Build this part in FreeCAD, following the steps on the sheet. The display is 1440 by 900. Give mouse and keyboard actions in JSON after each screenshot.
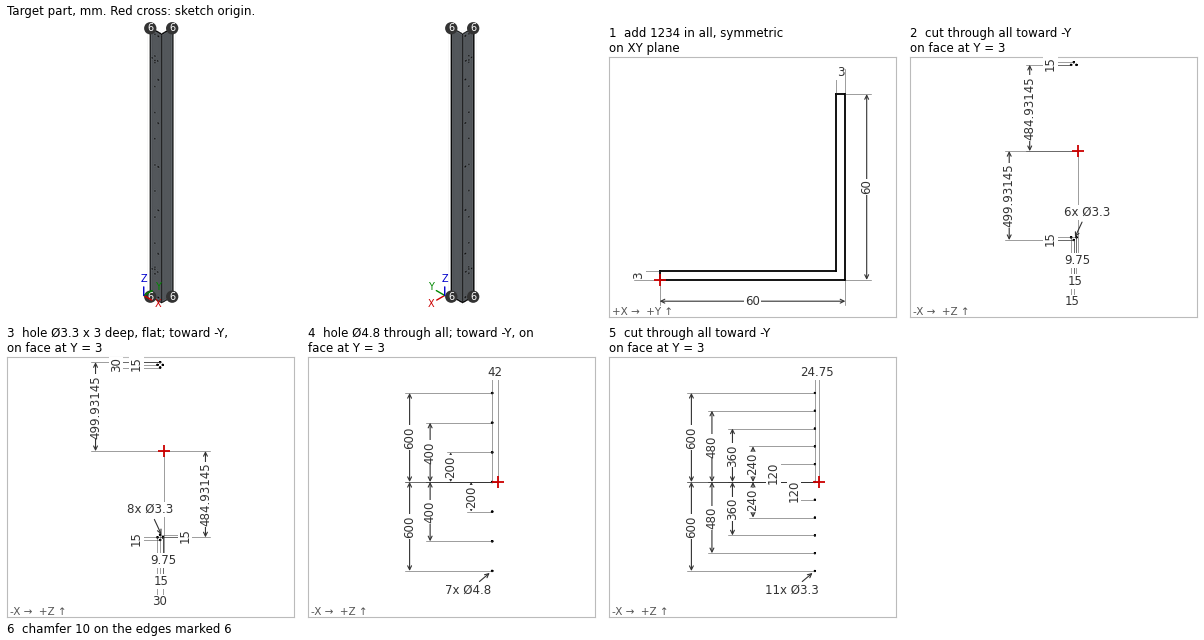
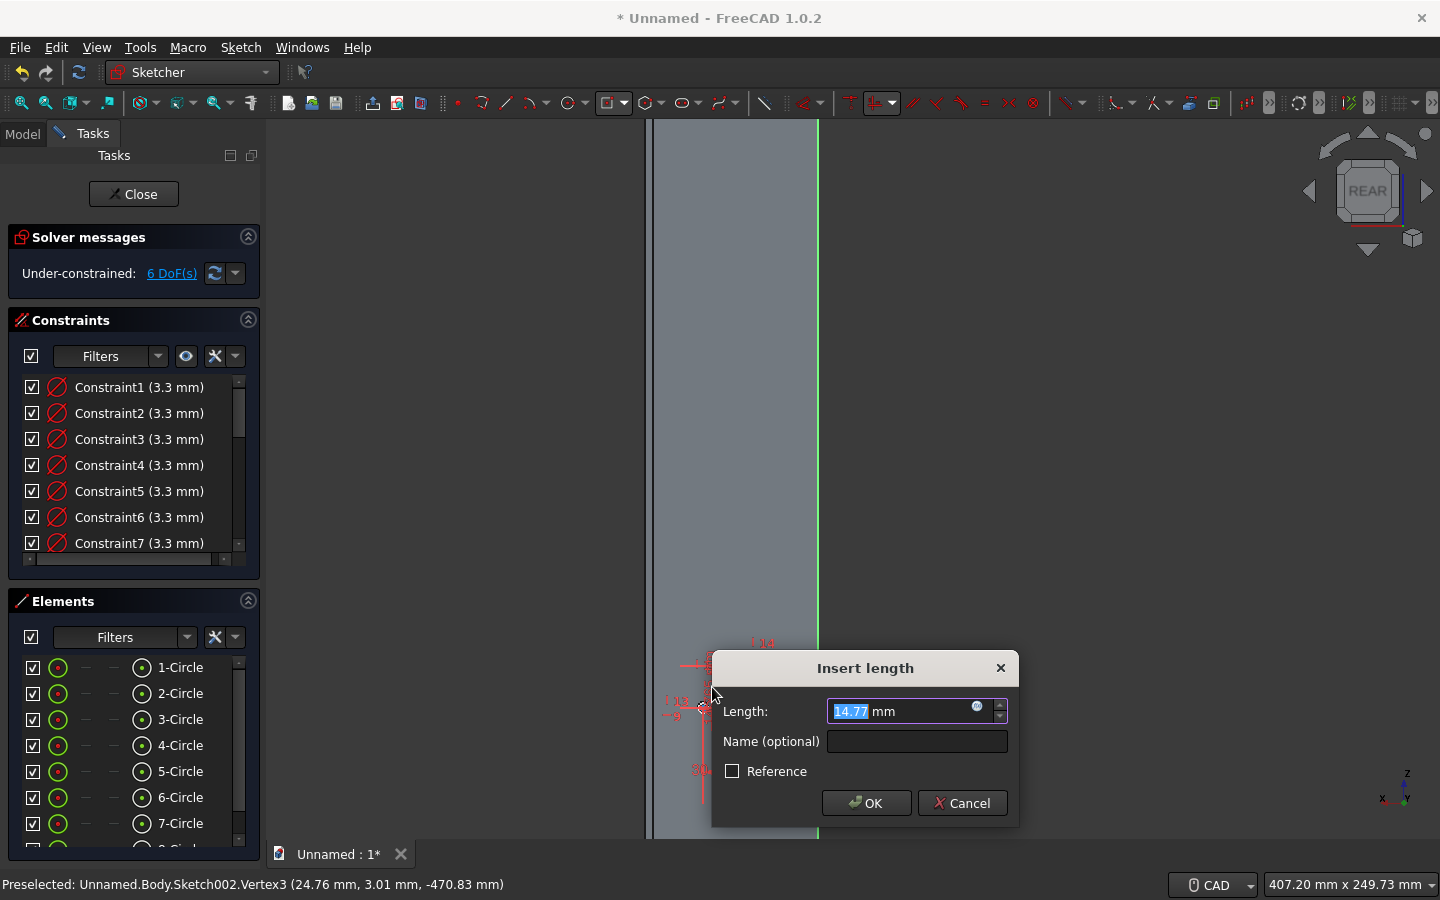
{"action": "type", "text": "15"}
{"action": "key", "text": "Return"}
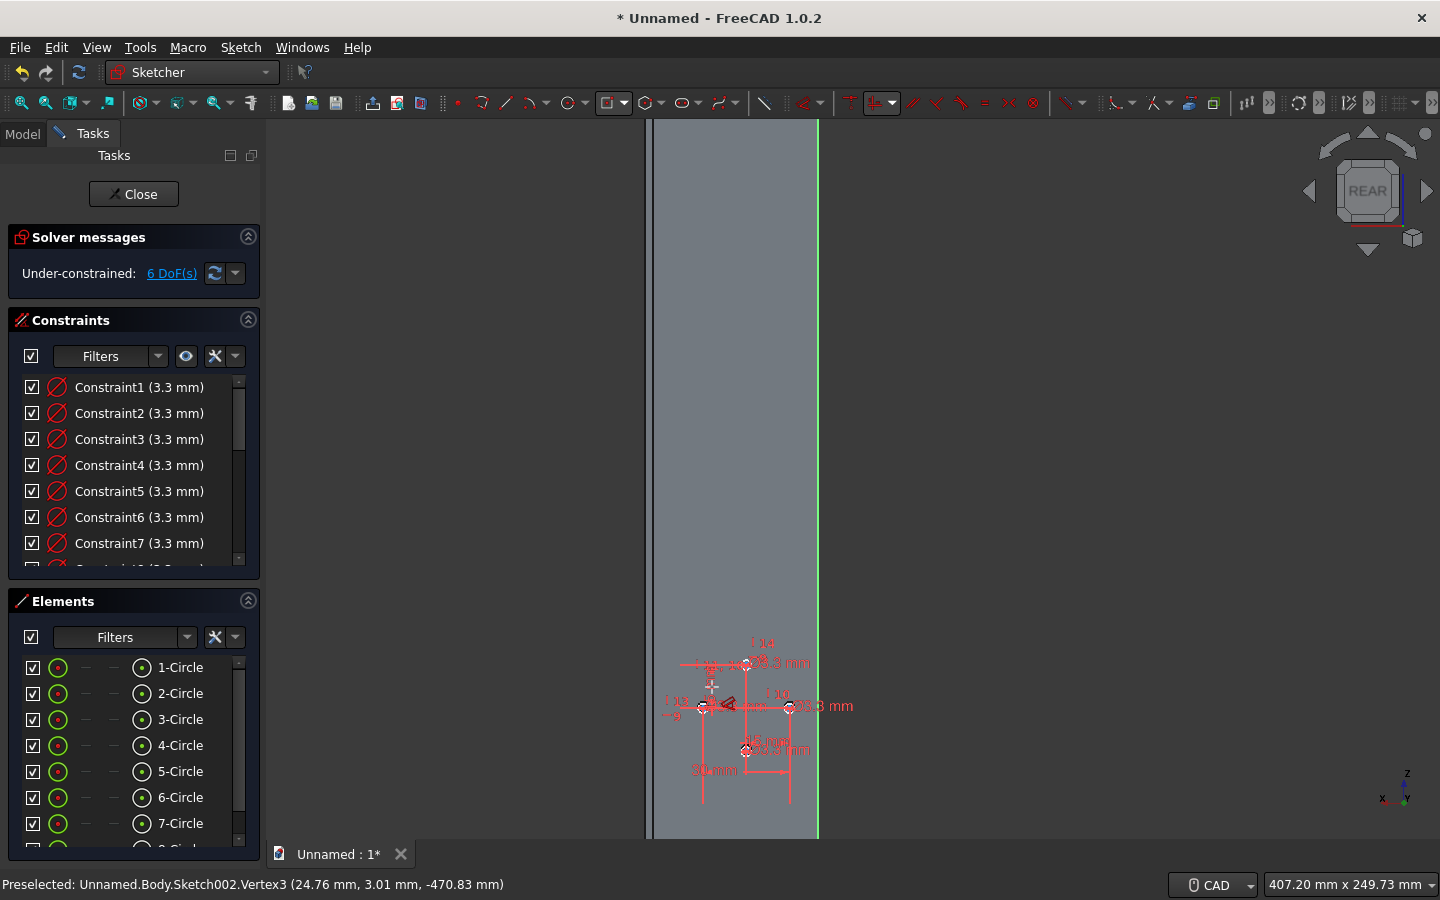
{"action": "left_click", "coordinate": [790, 708]}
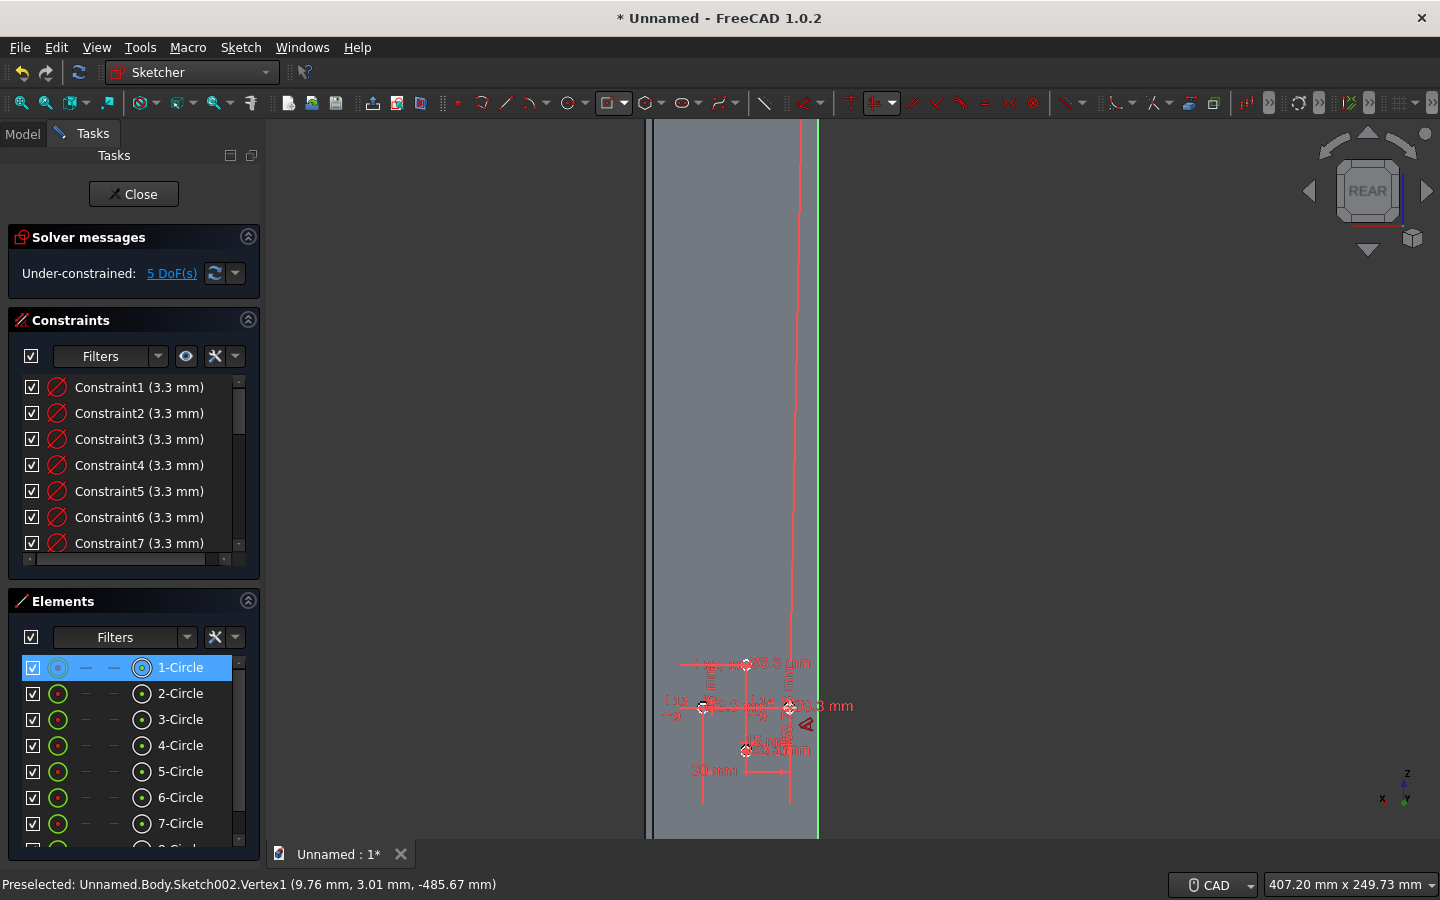
{"action": "left_click", "coordinate": [746, 752]}
{"action": "left_click", "coordinate": [848, 730]}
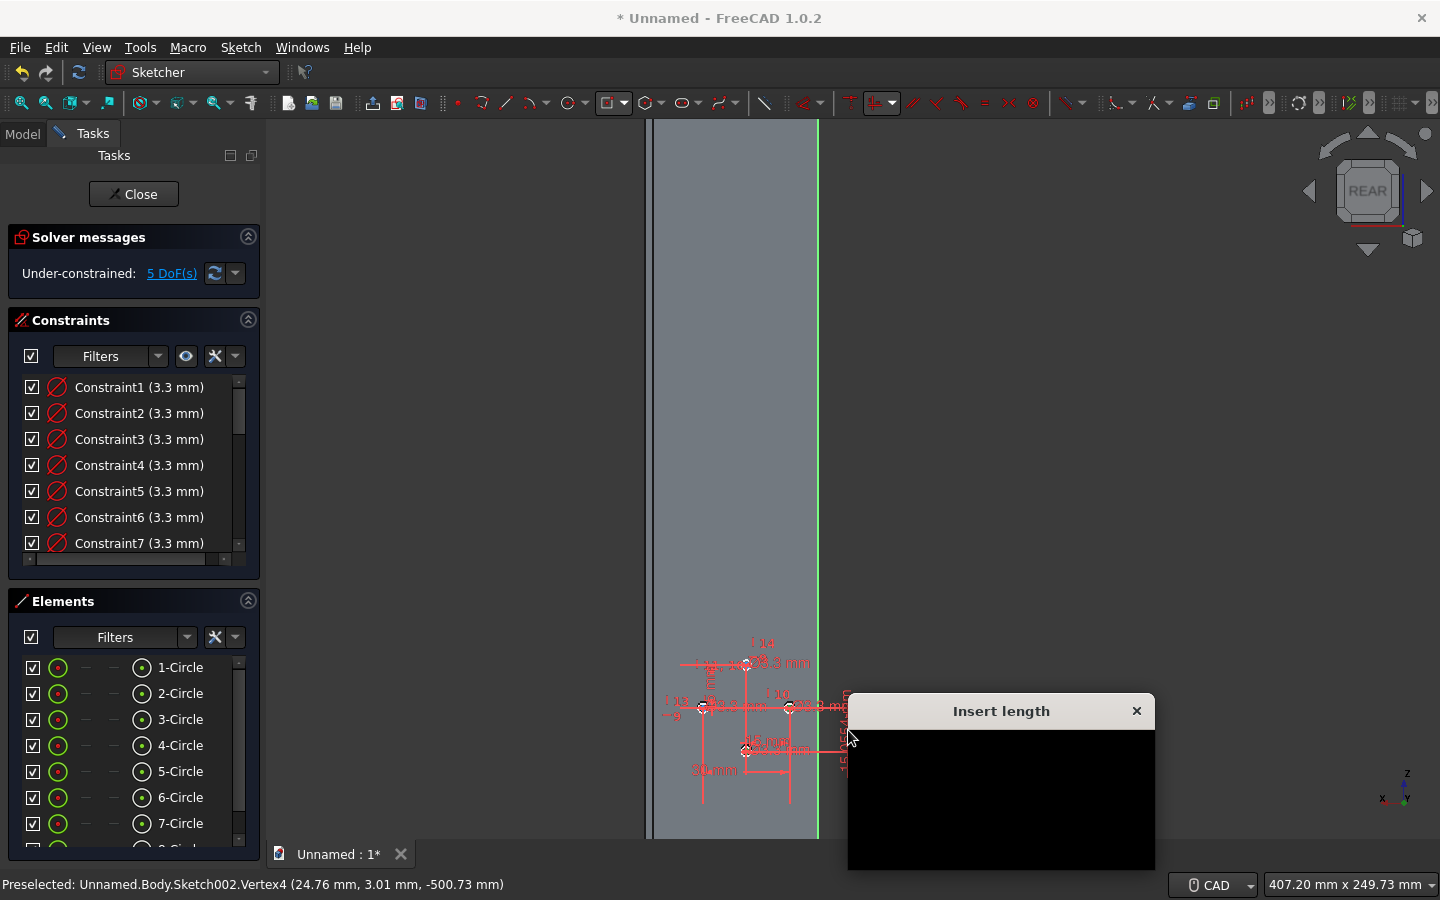
{"action": "type", "text": "15"}
{"action": "key", "text": "Return"}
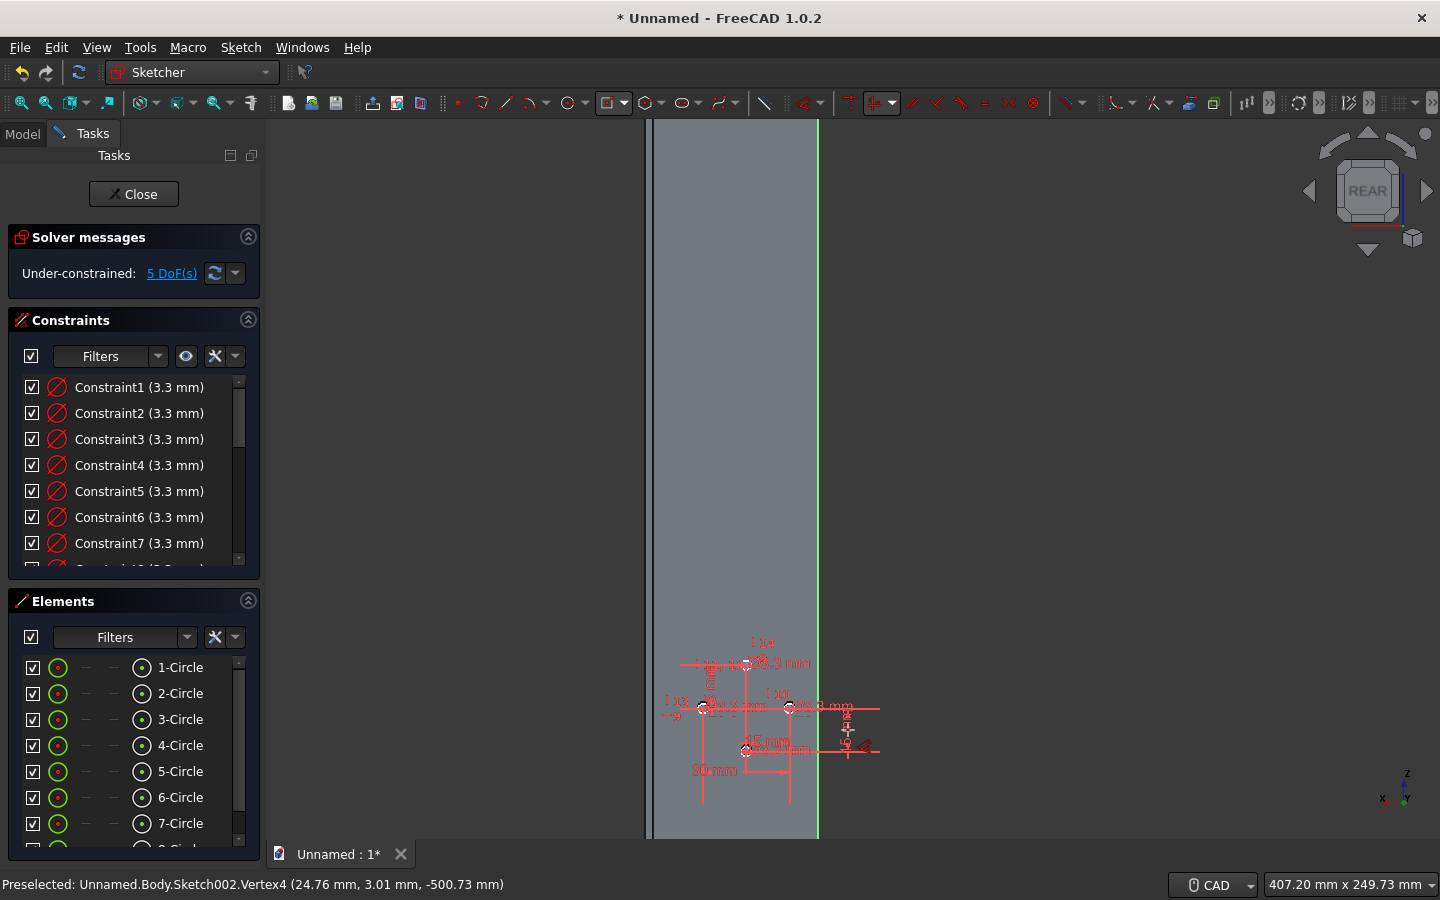
{"action": "scroll", "coordinate": [790, 711], "scroll_direction": "down", "scroll_amount": 9}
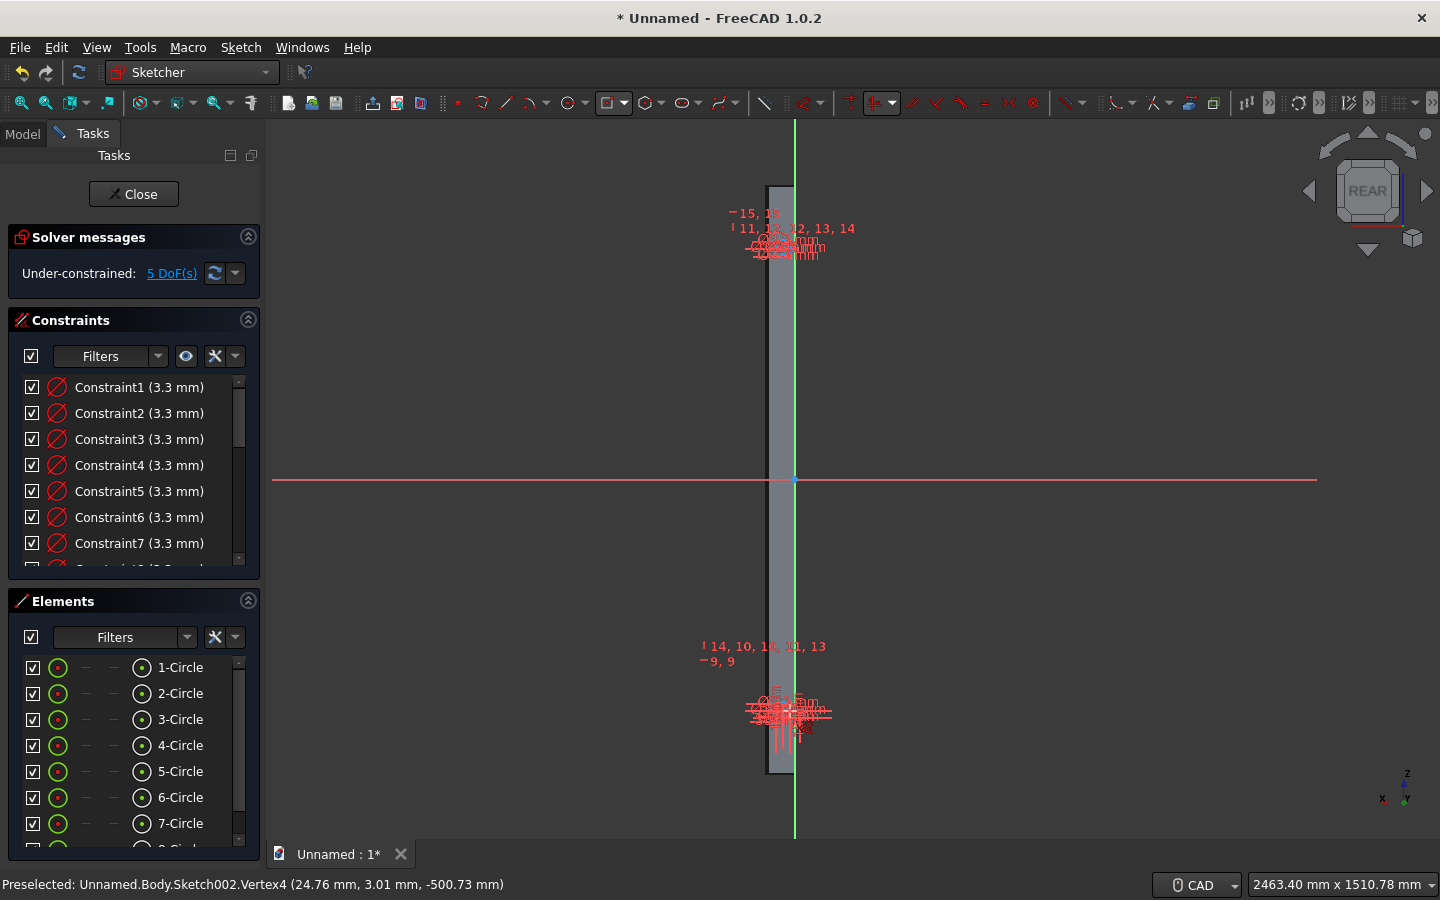
{"action": "scroll", "coordinate": [783, 242], "scroll_direction": "up", "scroll_amount": 6}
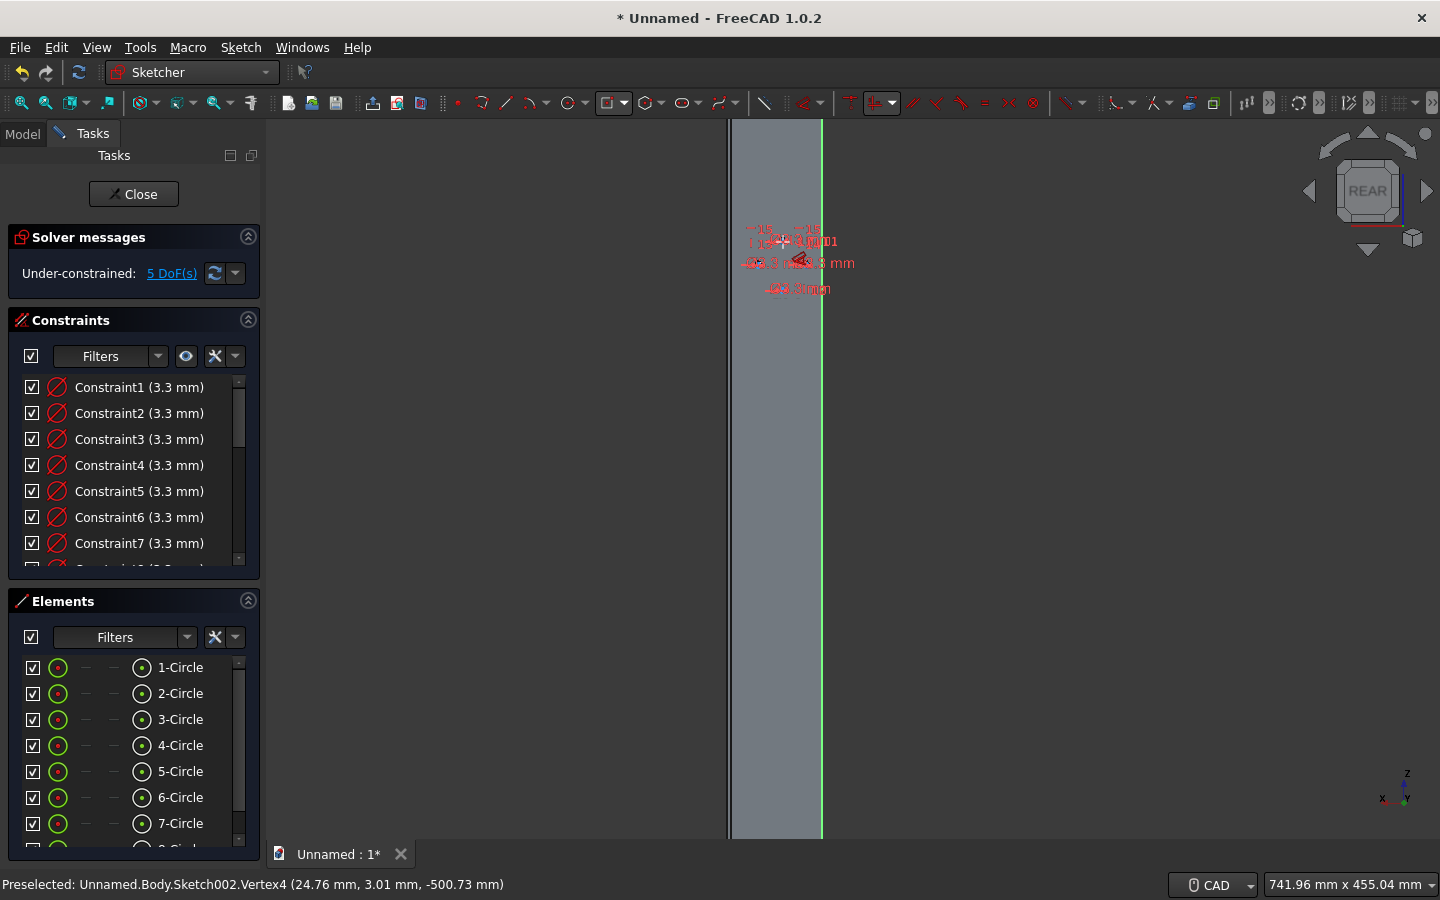
{"action": "left_click", "coordinate": [782, 242]}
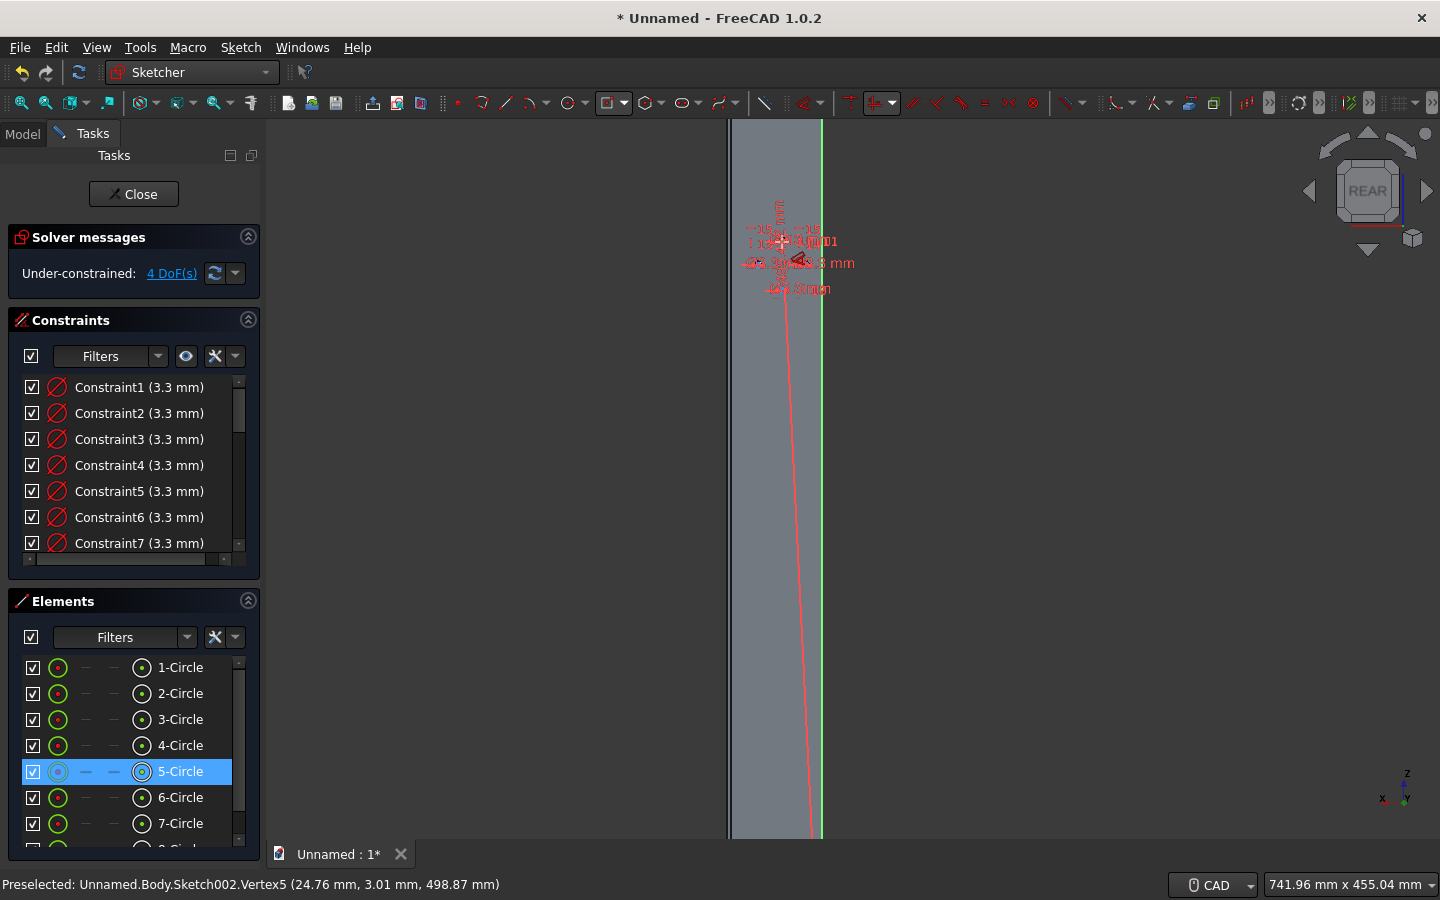
{"action": "left_click", "coordinate": [782, 291]}
{"action": "left_click", "coordinate": [748, 277]}